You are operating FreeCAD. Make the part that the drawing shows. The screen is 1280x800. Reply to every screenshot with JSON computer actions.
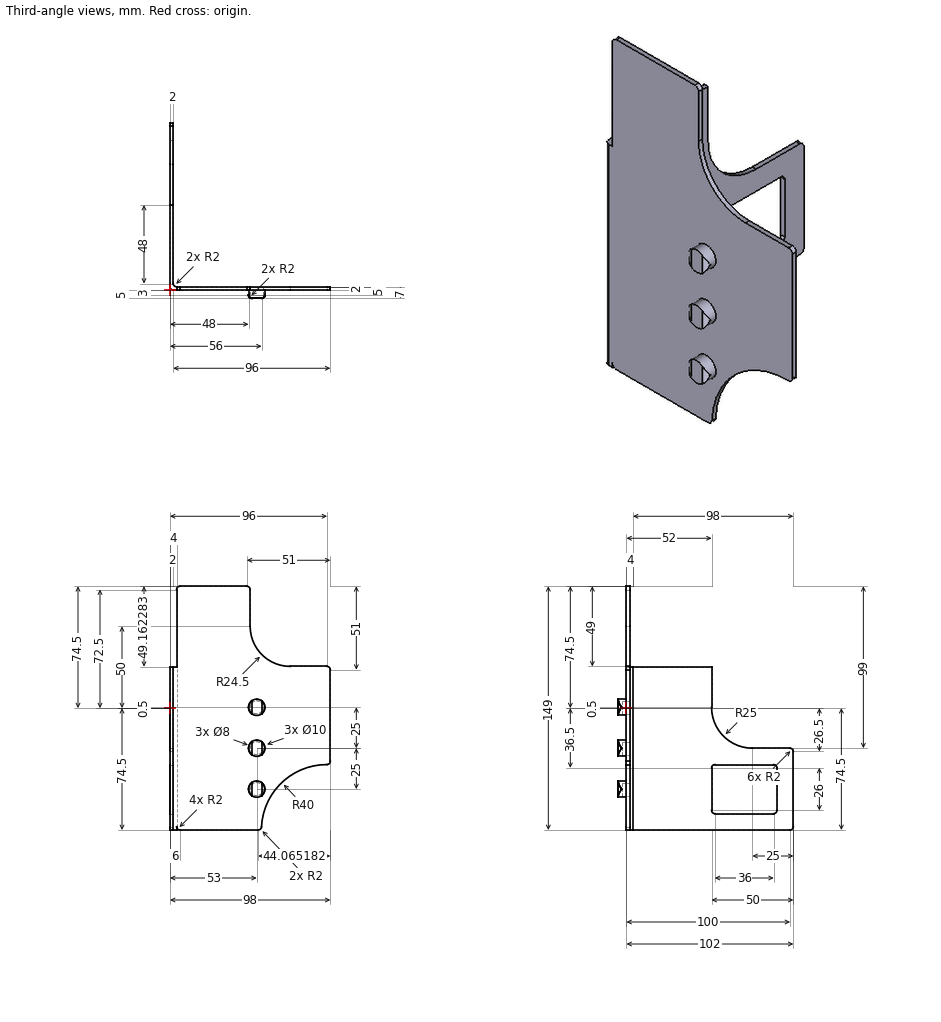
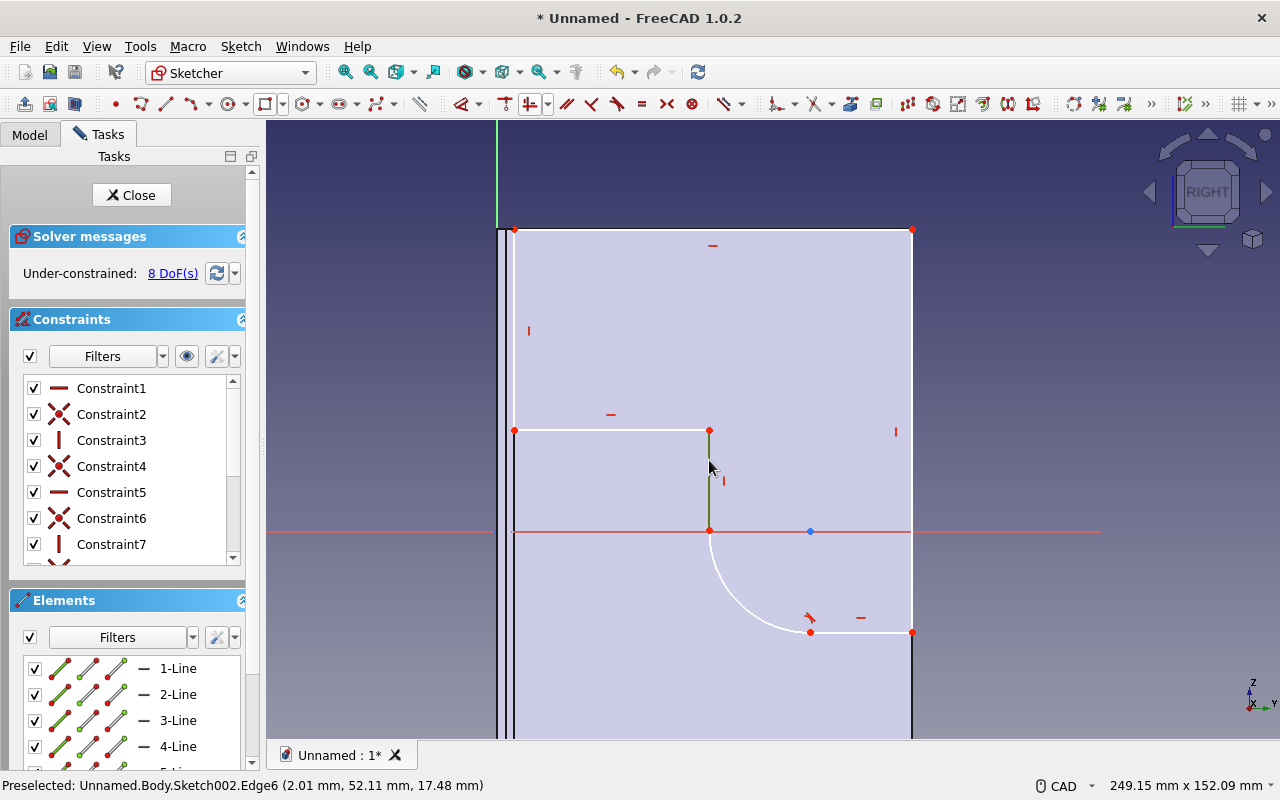
{"action": "left_click", "coordinate": [720, 577]}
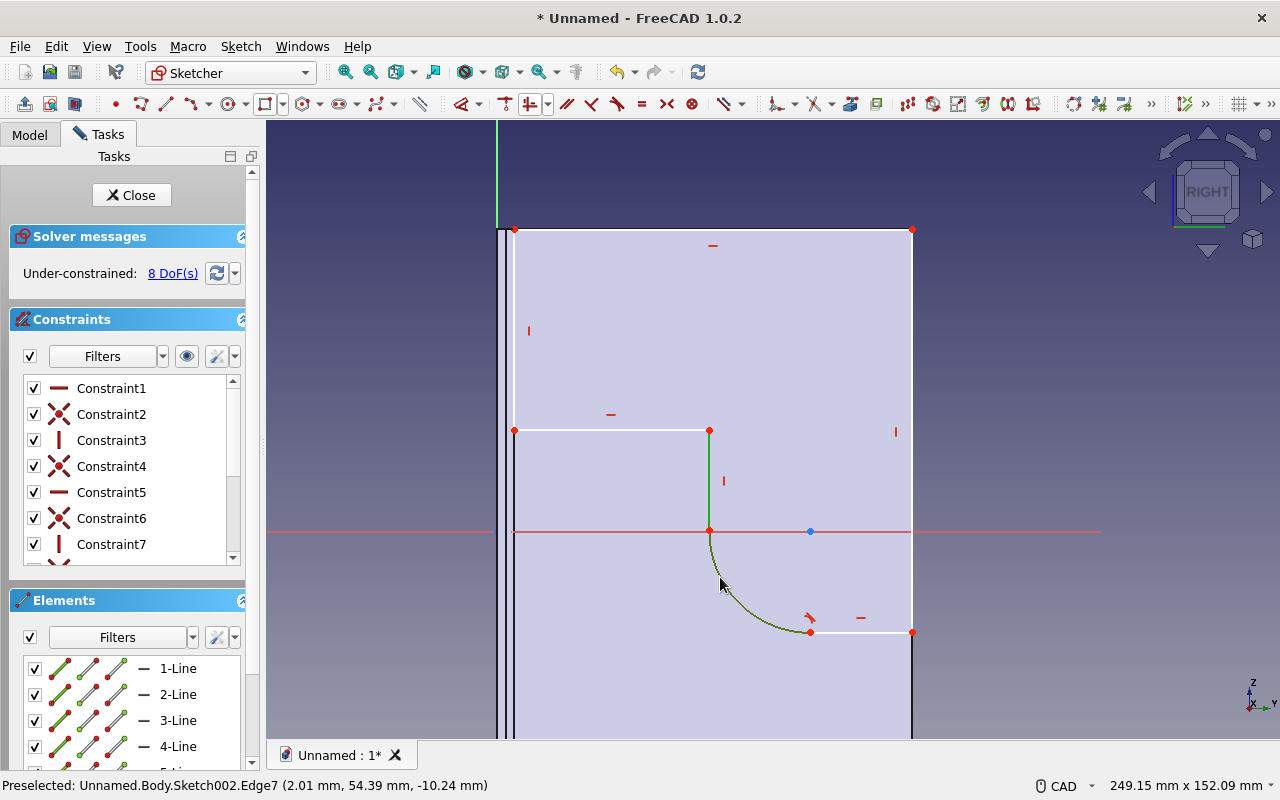
{"action": "left_click", "coordinate": [617, 104]}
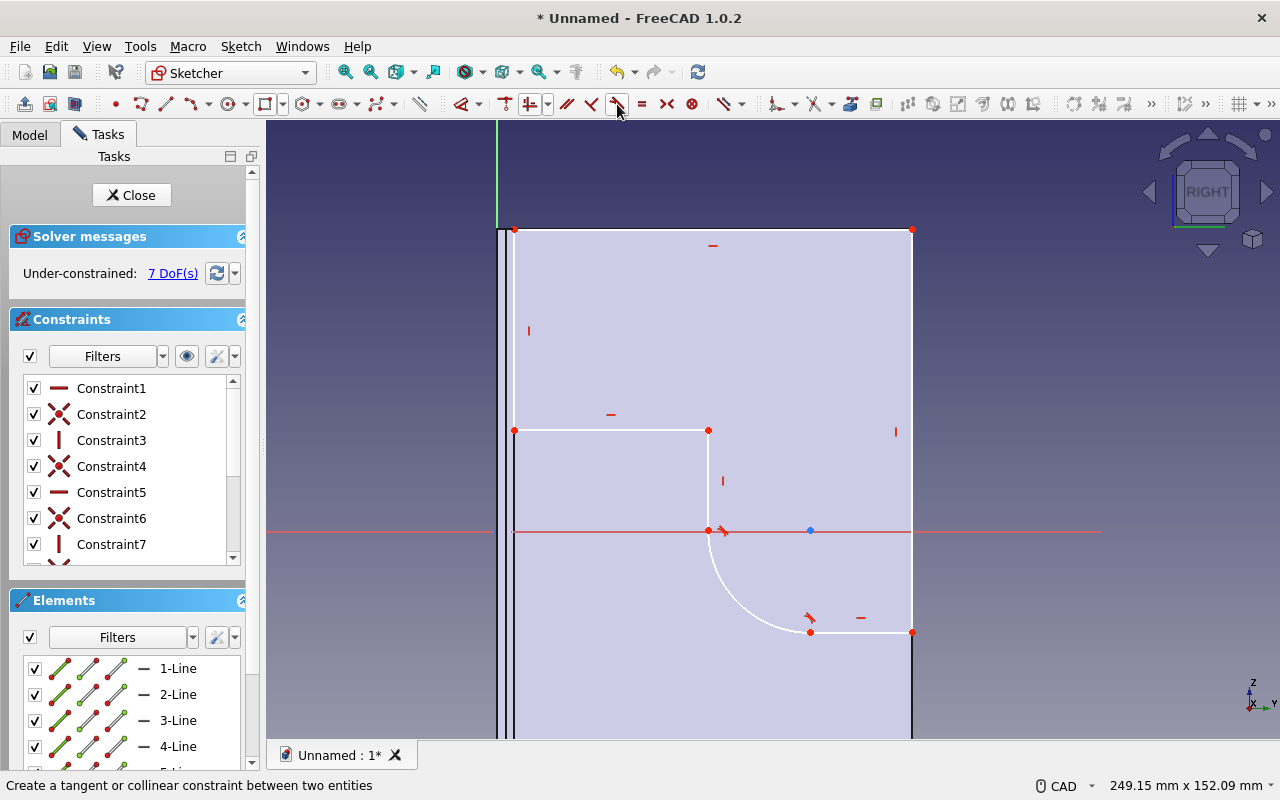
{"action": "left_click", "coordinate": [719, 577]}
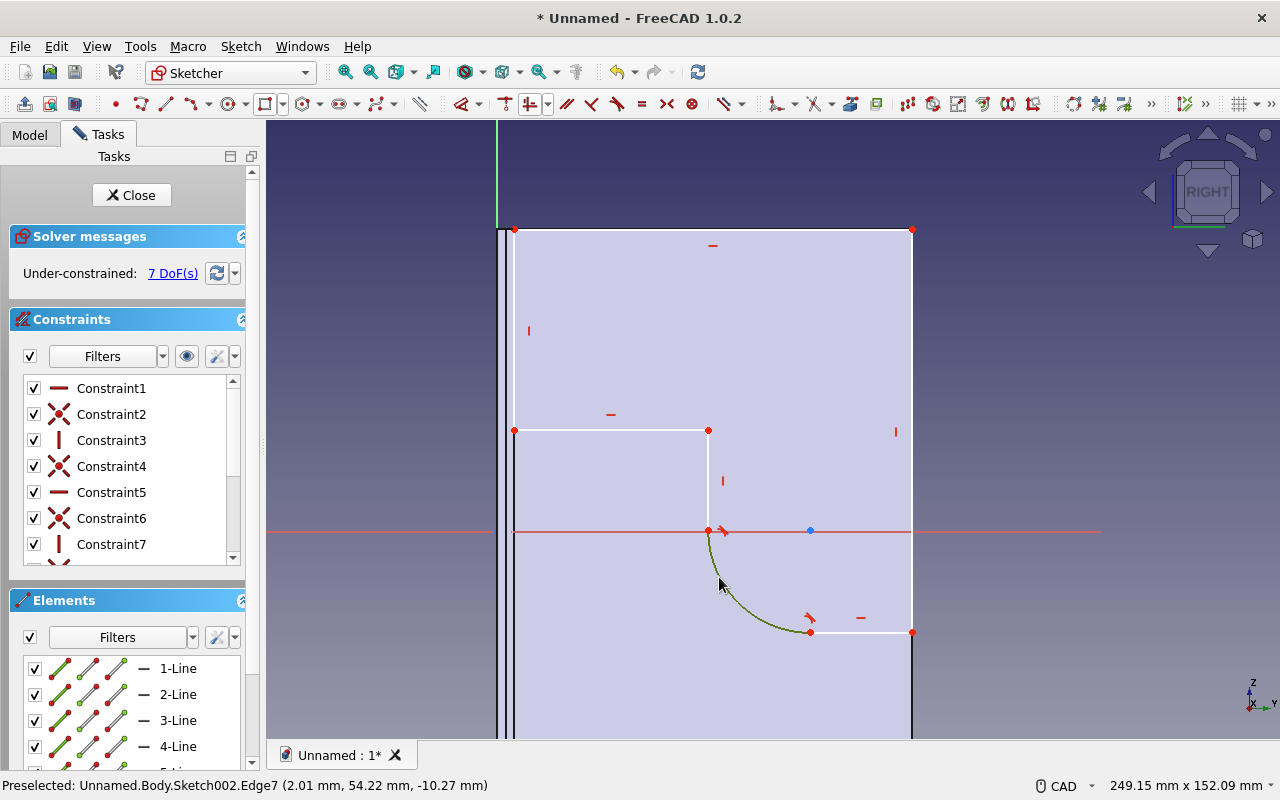
{"action": "key", "text": "k r"}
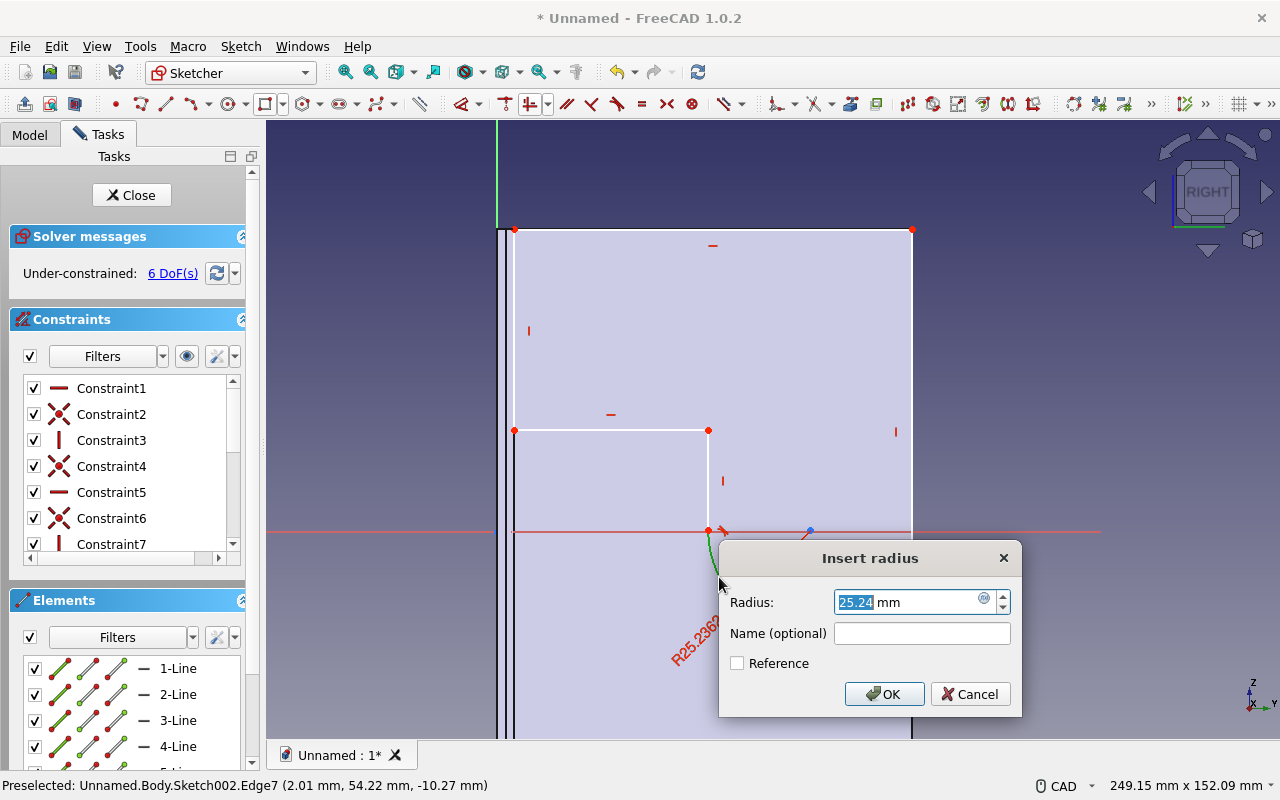
{"action": "type", "text": "25"}
{"action": "key", "text": "Return"}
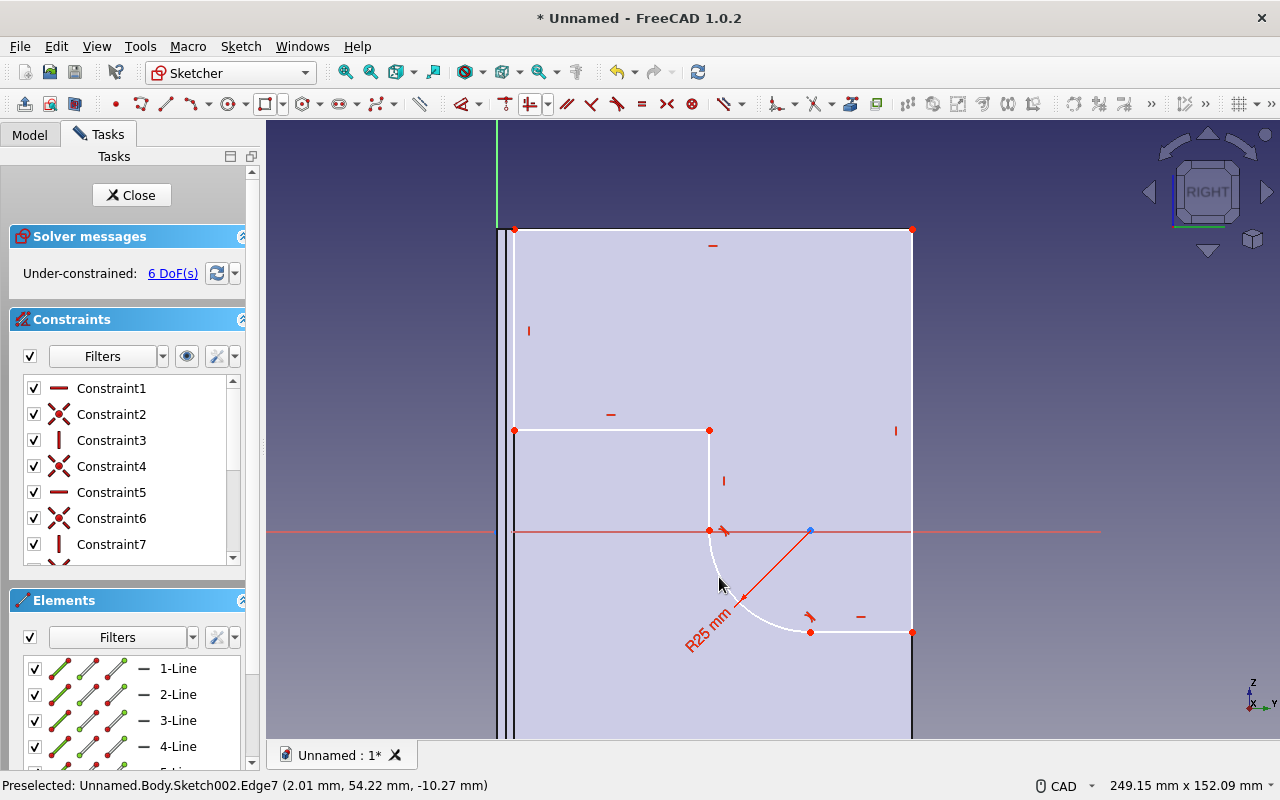
{"action": "left_click", "coordinate": [841, 632]}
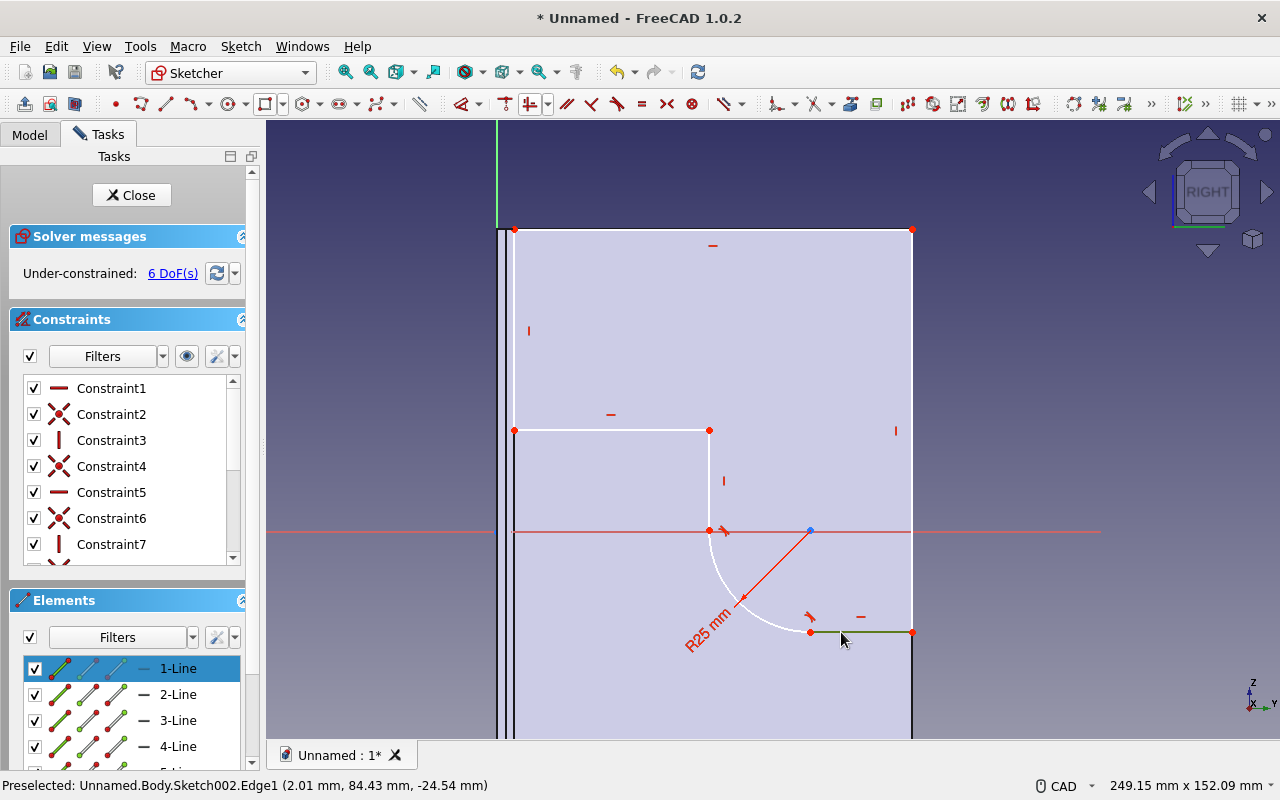
{"action": "key", "text": "l"}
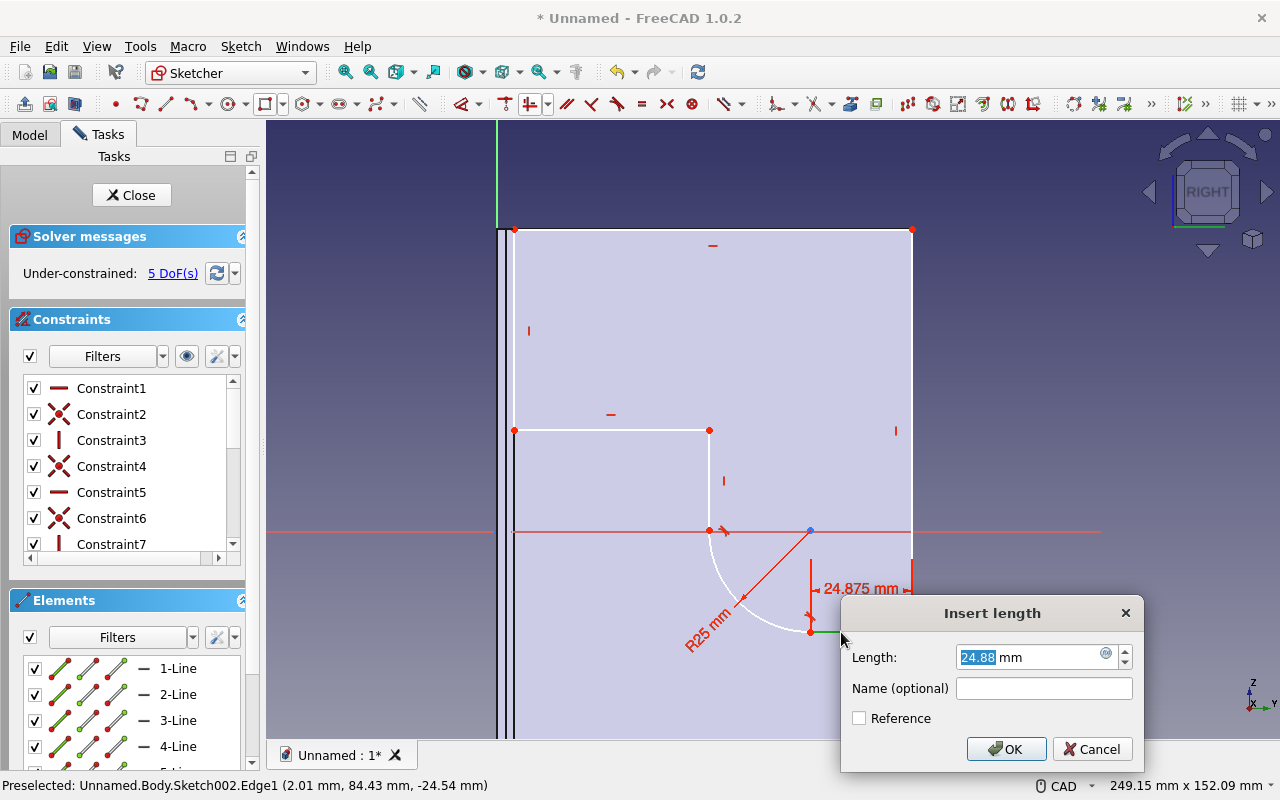
{"action": "type", "text": "25"}
{"action": "key", "text": "Return"}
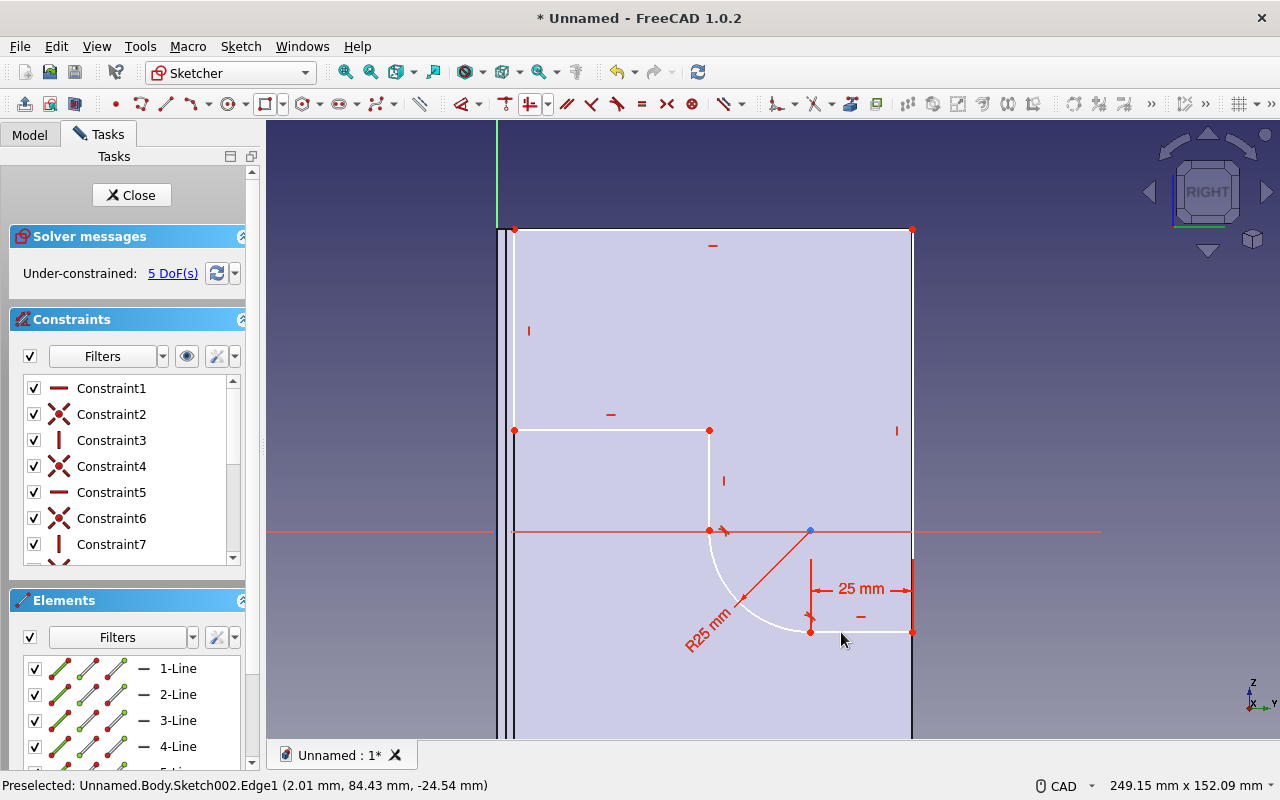
{"action": "left_click", "coordinate": [913, 511]}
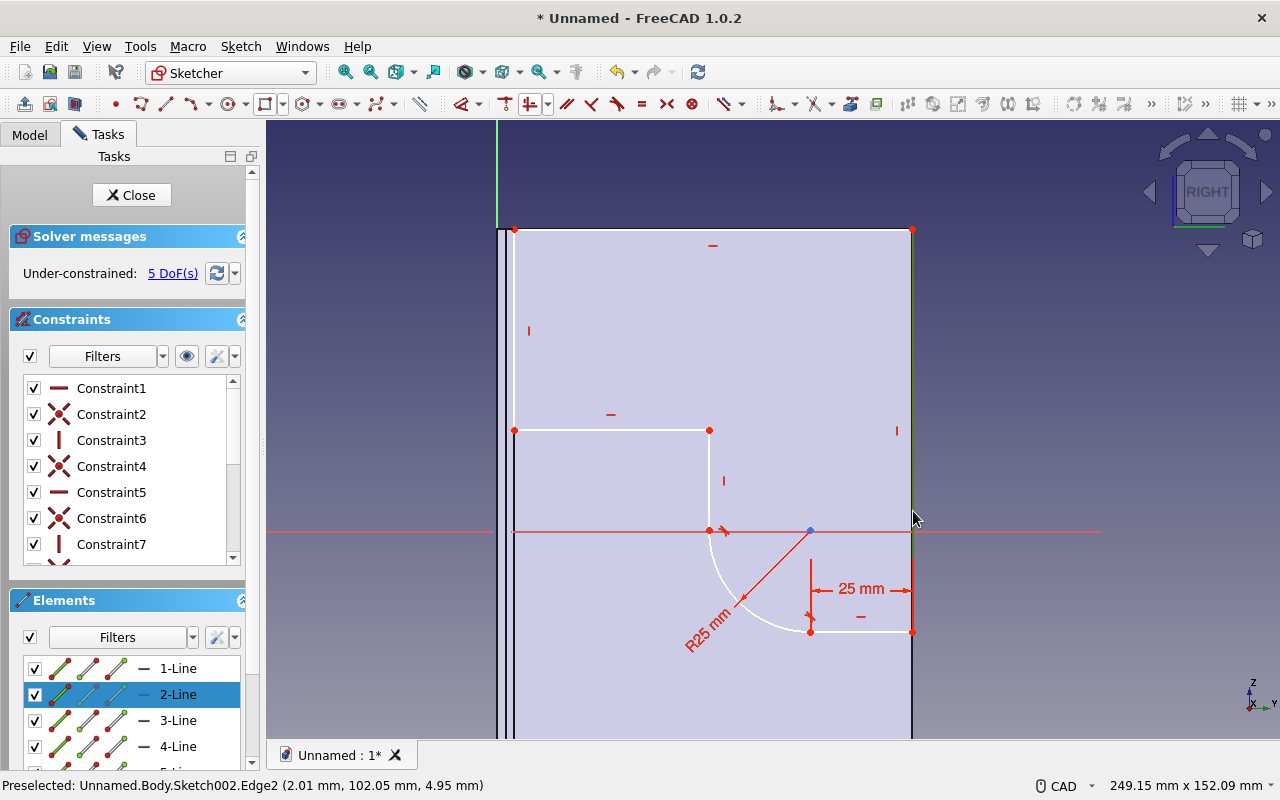
{"action": "key", "text": "i"}